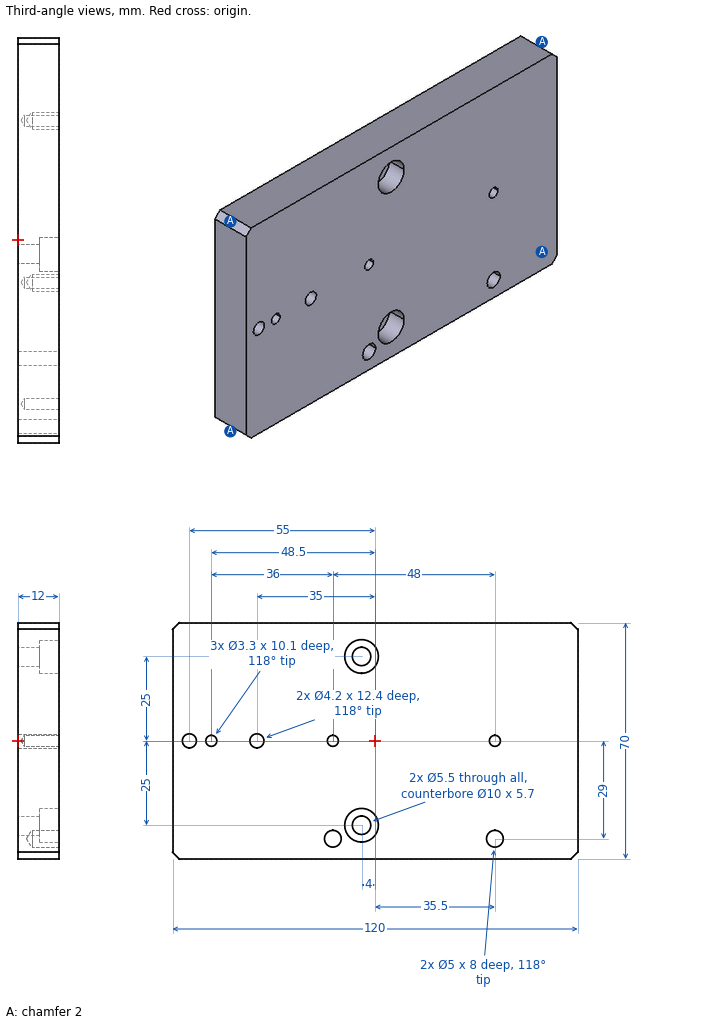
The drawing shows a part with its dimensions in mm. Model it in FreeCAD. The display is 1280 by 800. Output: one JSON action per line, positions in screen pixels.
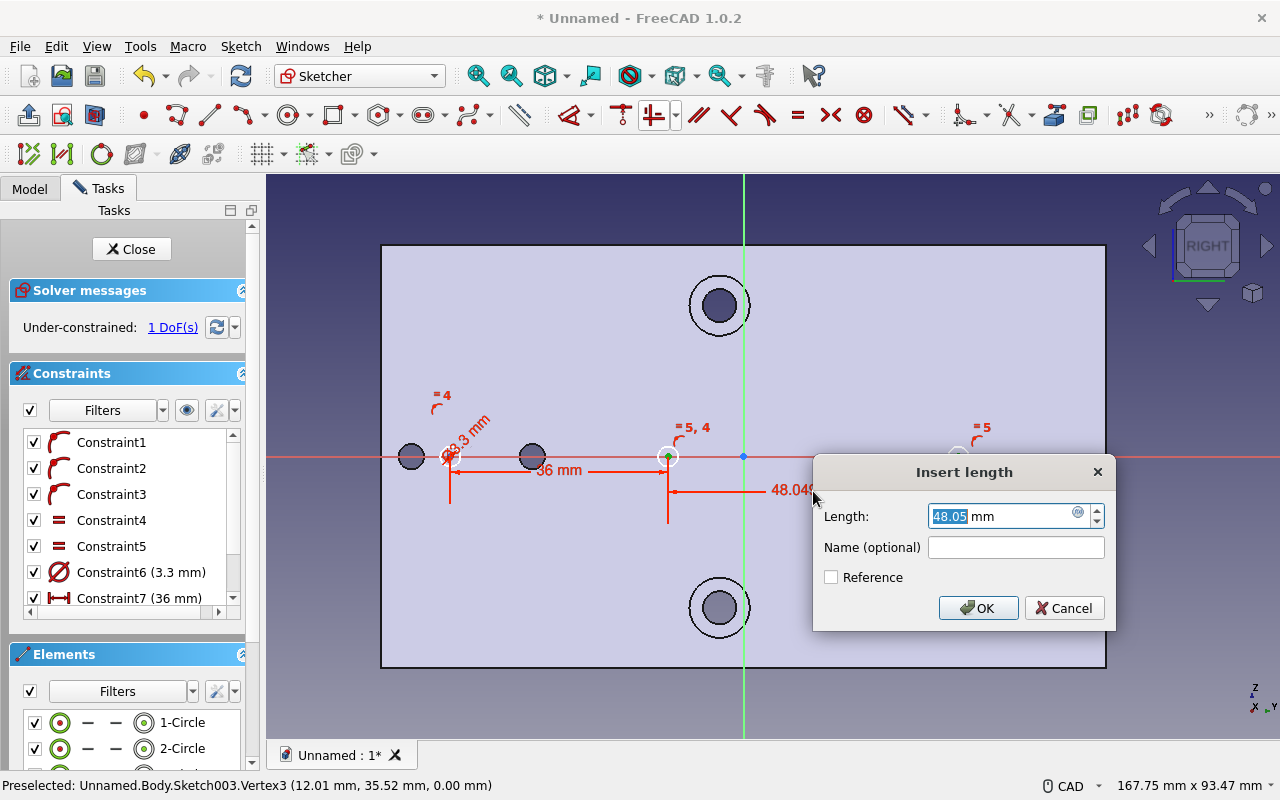
{"action": "type", "text": "48"}
{"action": "key", "text": "Return"}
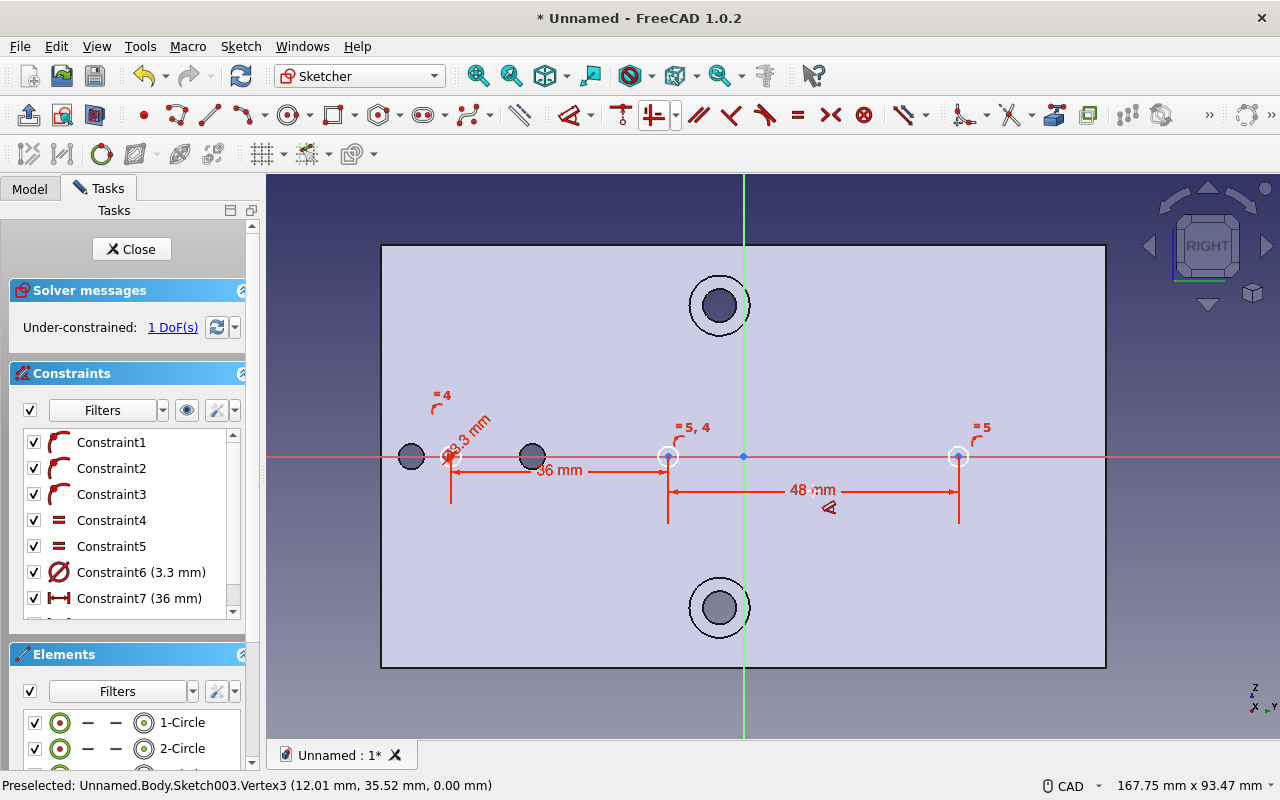
{"action": "left_click", "coordinate": [451, 457]}
{"action": "left_click", "coordinate": [665, 491]}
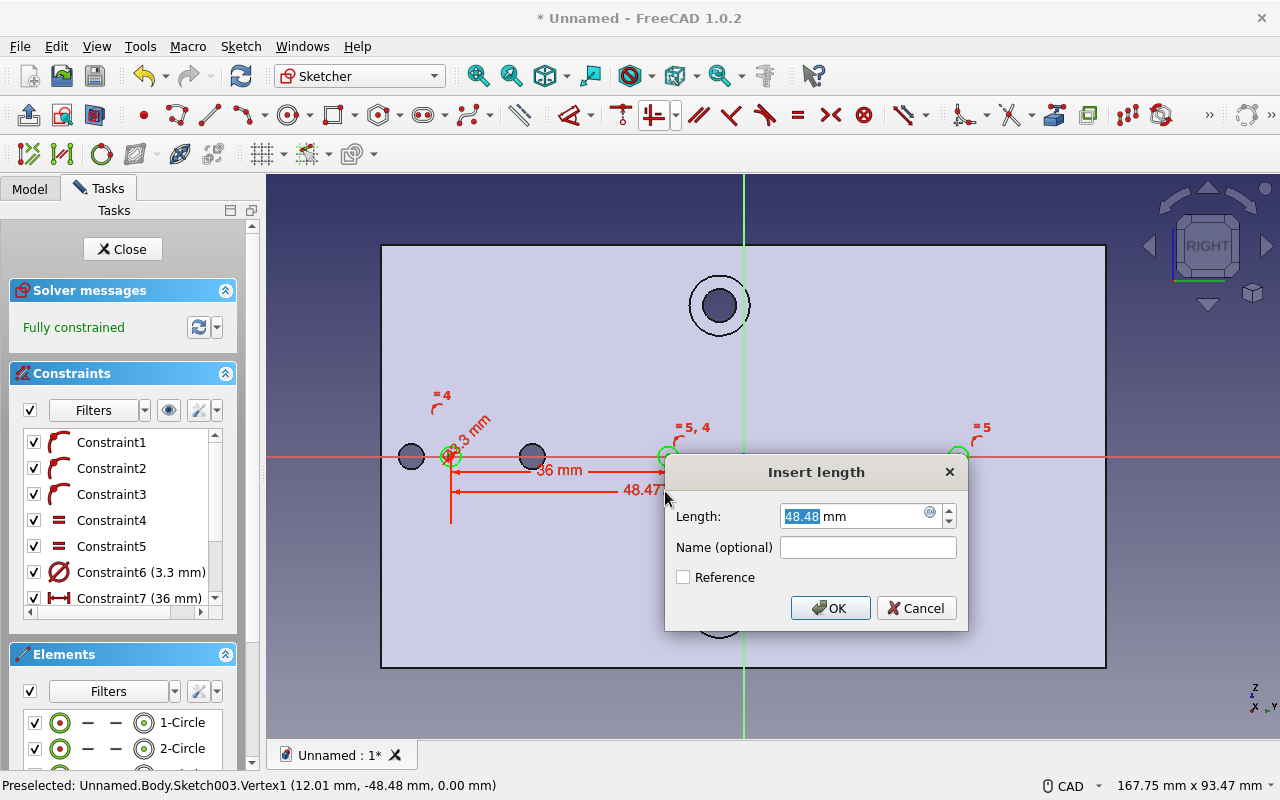
{"action": "type", "text": "48.5"}
{"action": "key", "text": "Return"}
{"action": "key", "text": "Escape"}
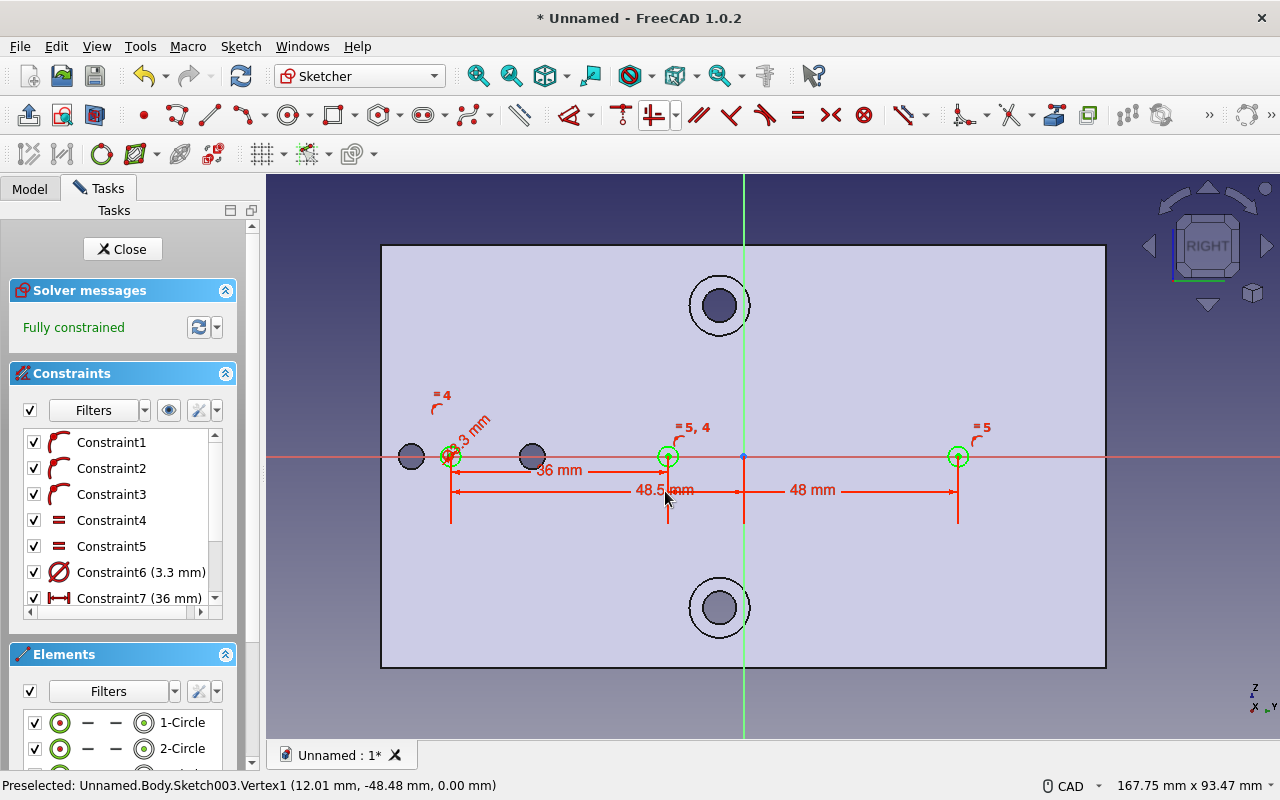
{"action": "left_click", "coordinate": [123, 249]}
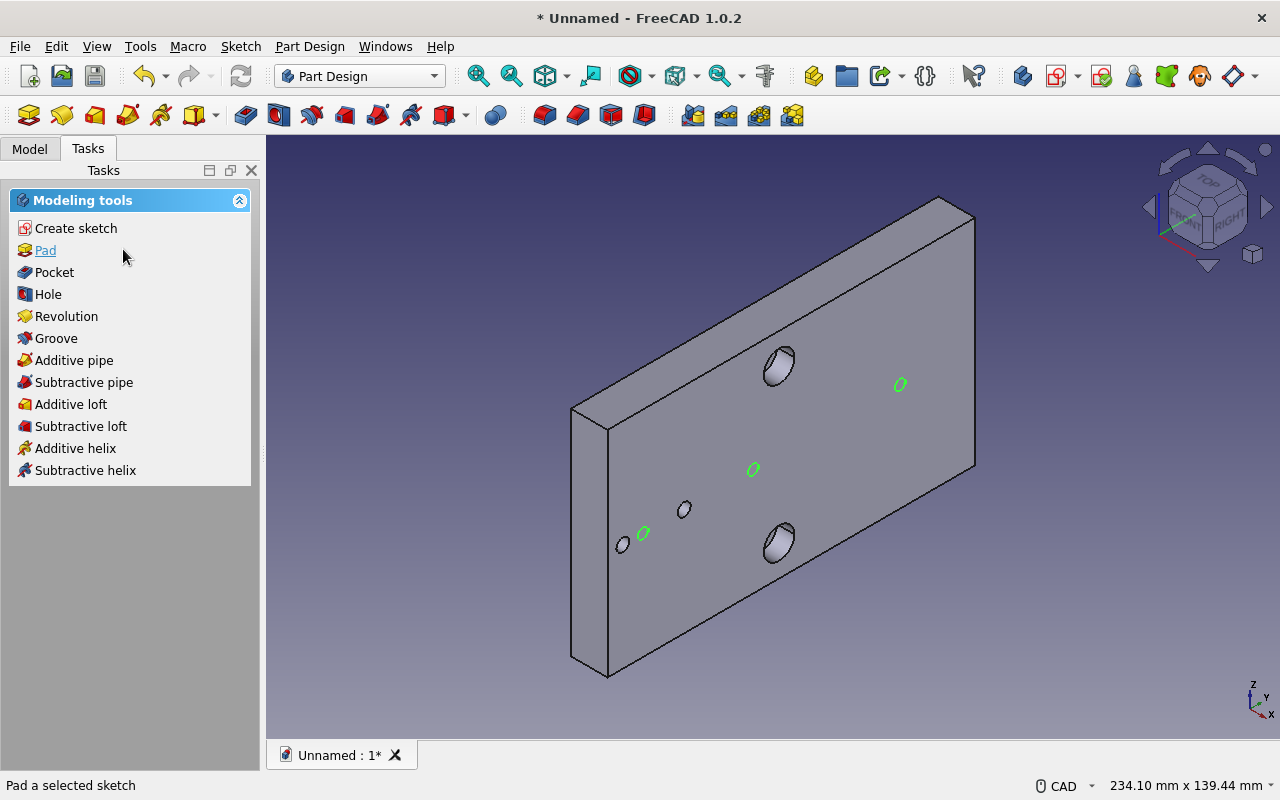
{"action": "left_click", "coordinate": [279, 116]}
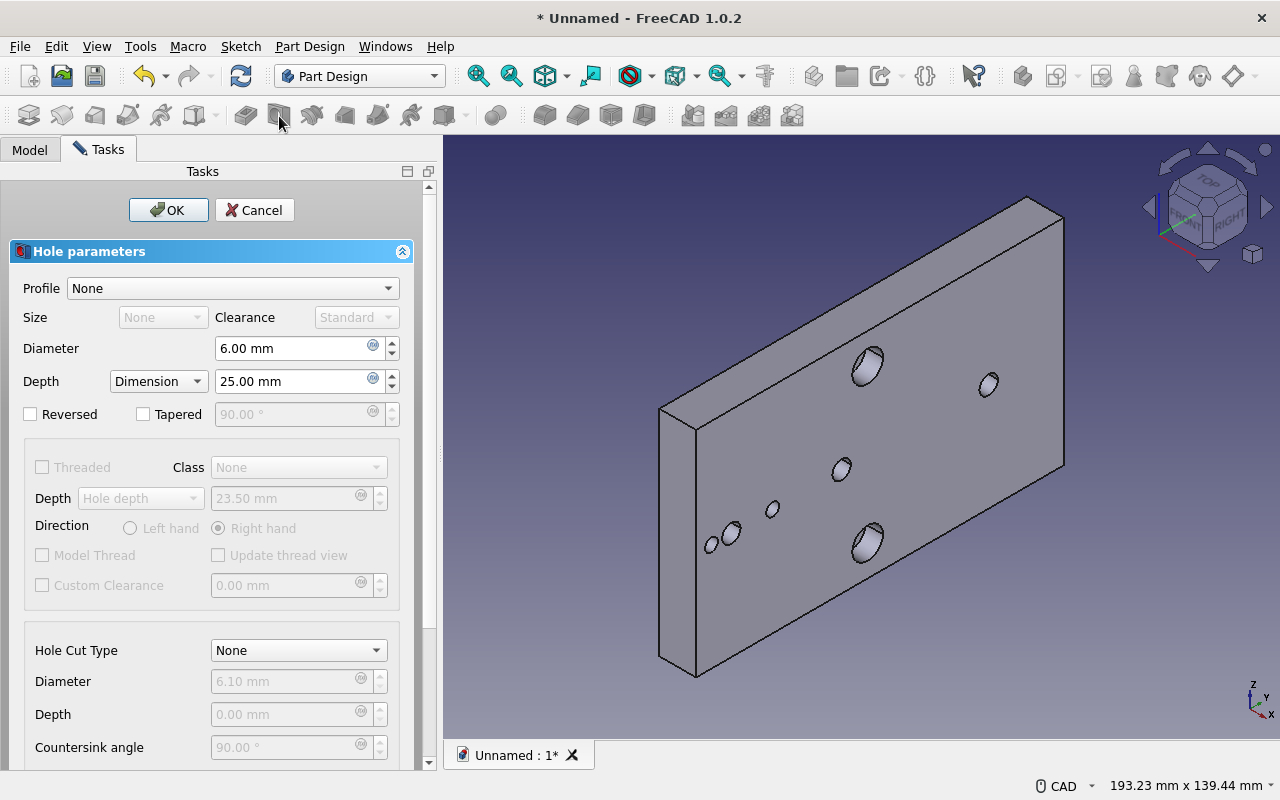
{"action": "triple_click", "coordinate": [300, 348]}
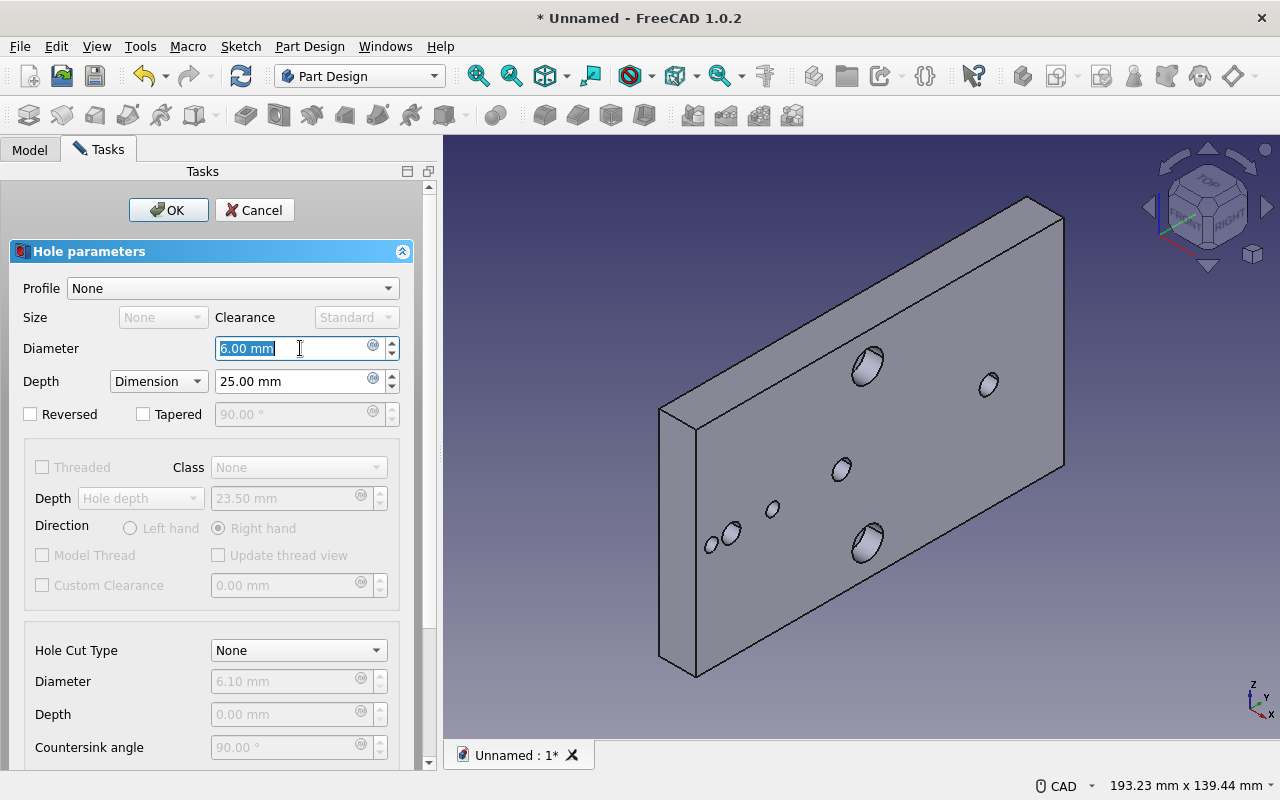
{"action": "type", "text": "3.3"}
{"action": "key", "text": "Tab"}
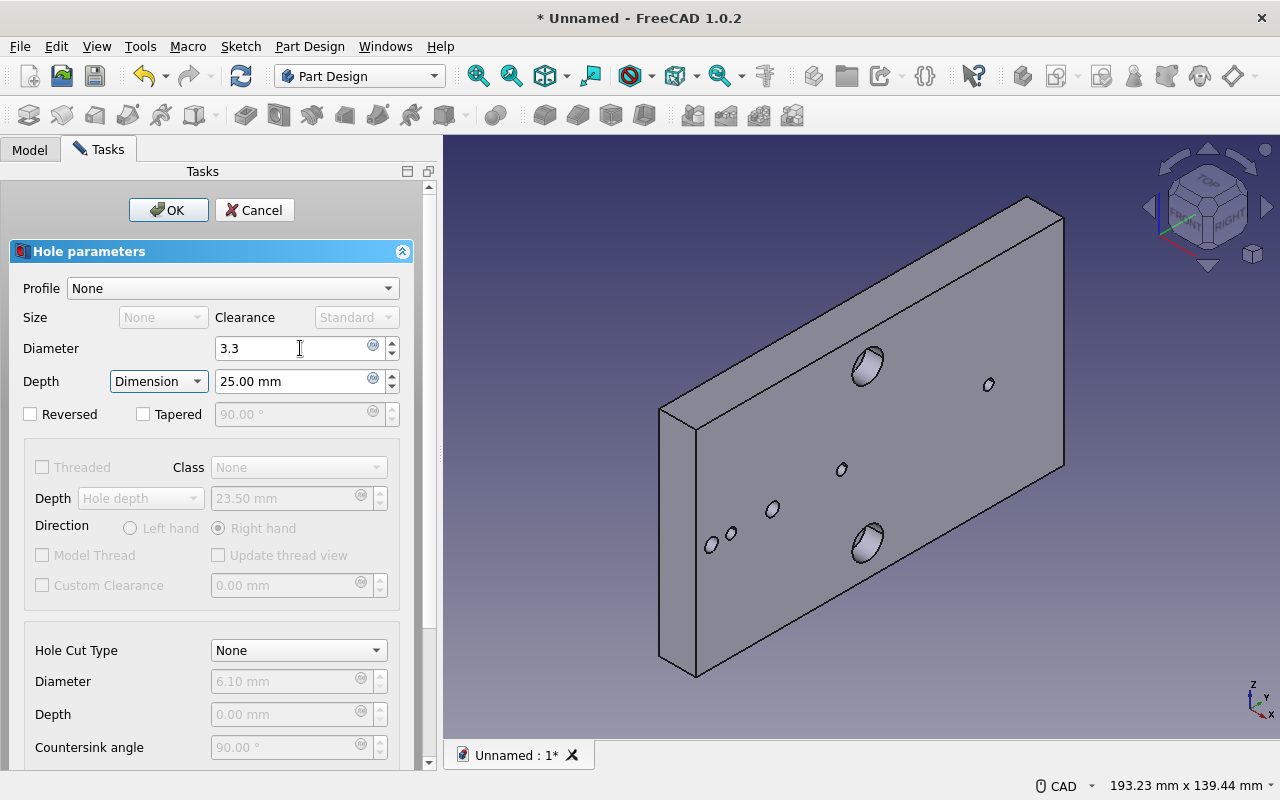
{"action": "triple_click", "coordinate": [300, 382]}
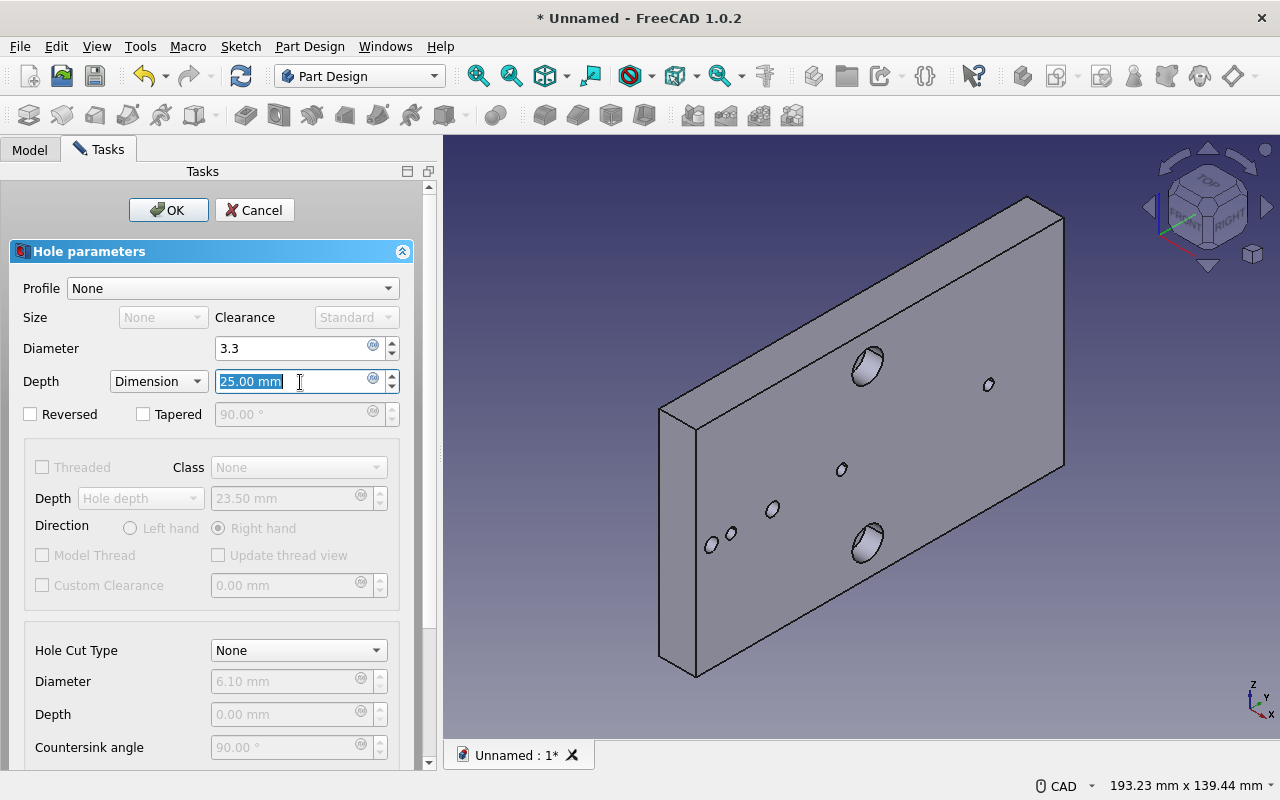
{"action": "type", "text": "10.1"}
{"action": "key", "text": "Tab"}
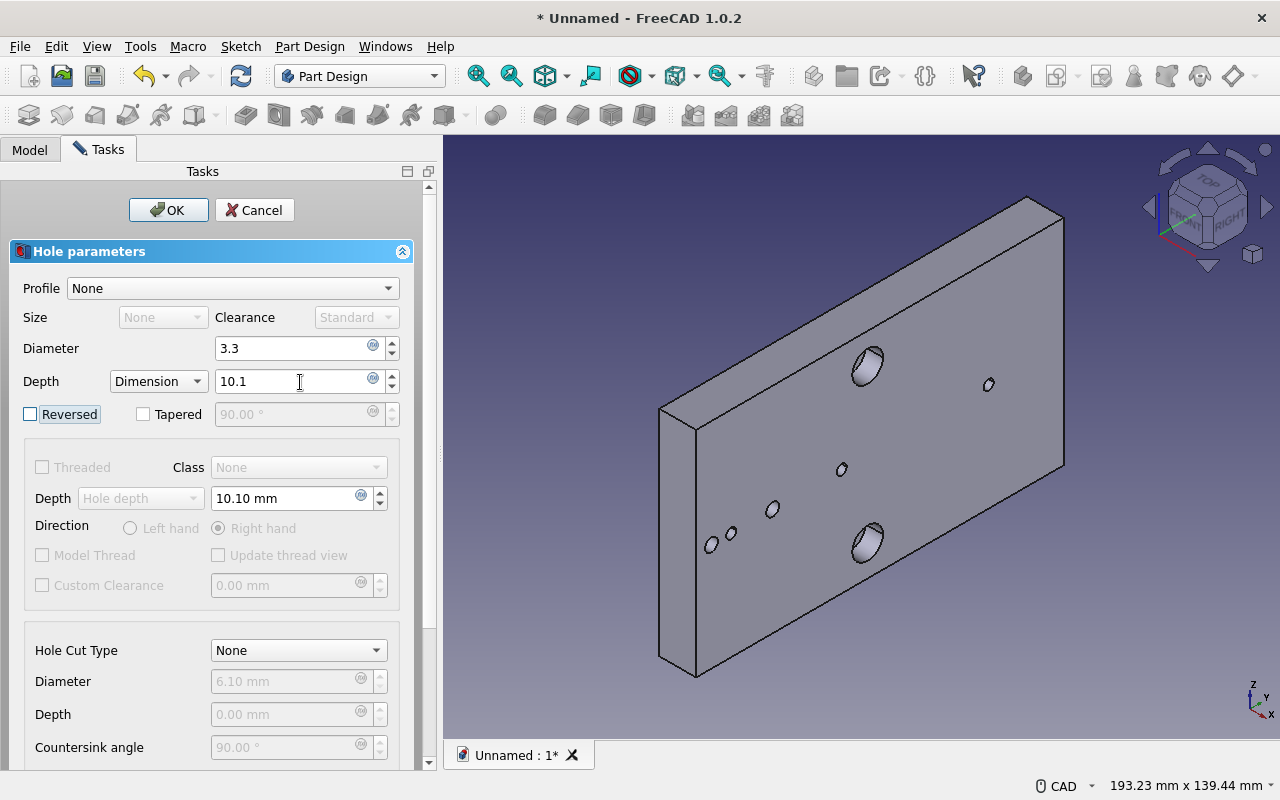
{"action": "left_click", "coordinate": [169, 210]}